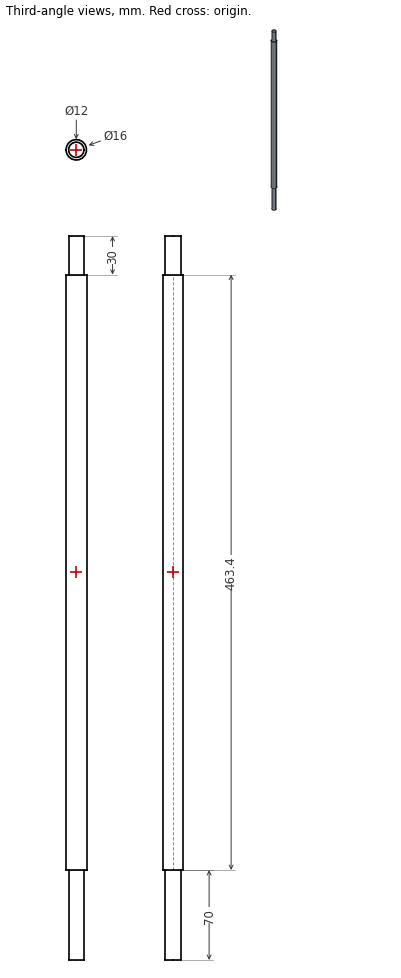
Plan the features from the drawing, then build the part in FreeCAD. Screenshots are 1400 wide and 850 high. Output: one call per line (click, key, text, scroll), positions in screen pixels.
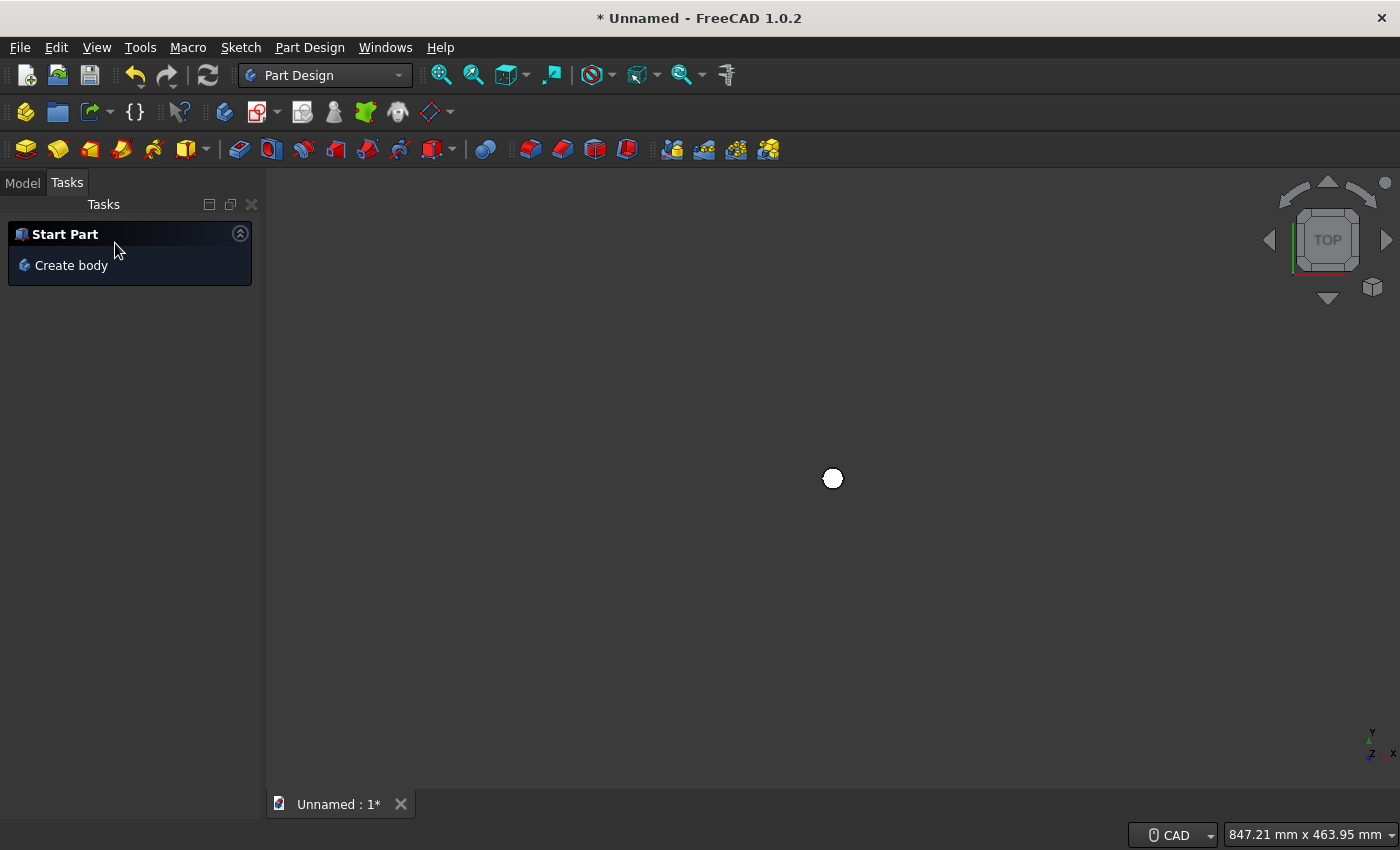
key(v)
key(f)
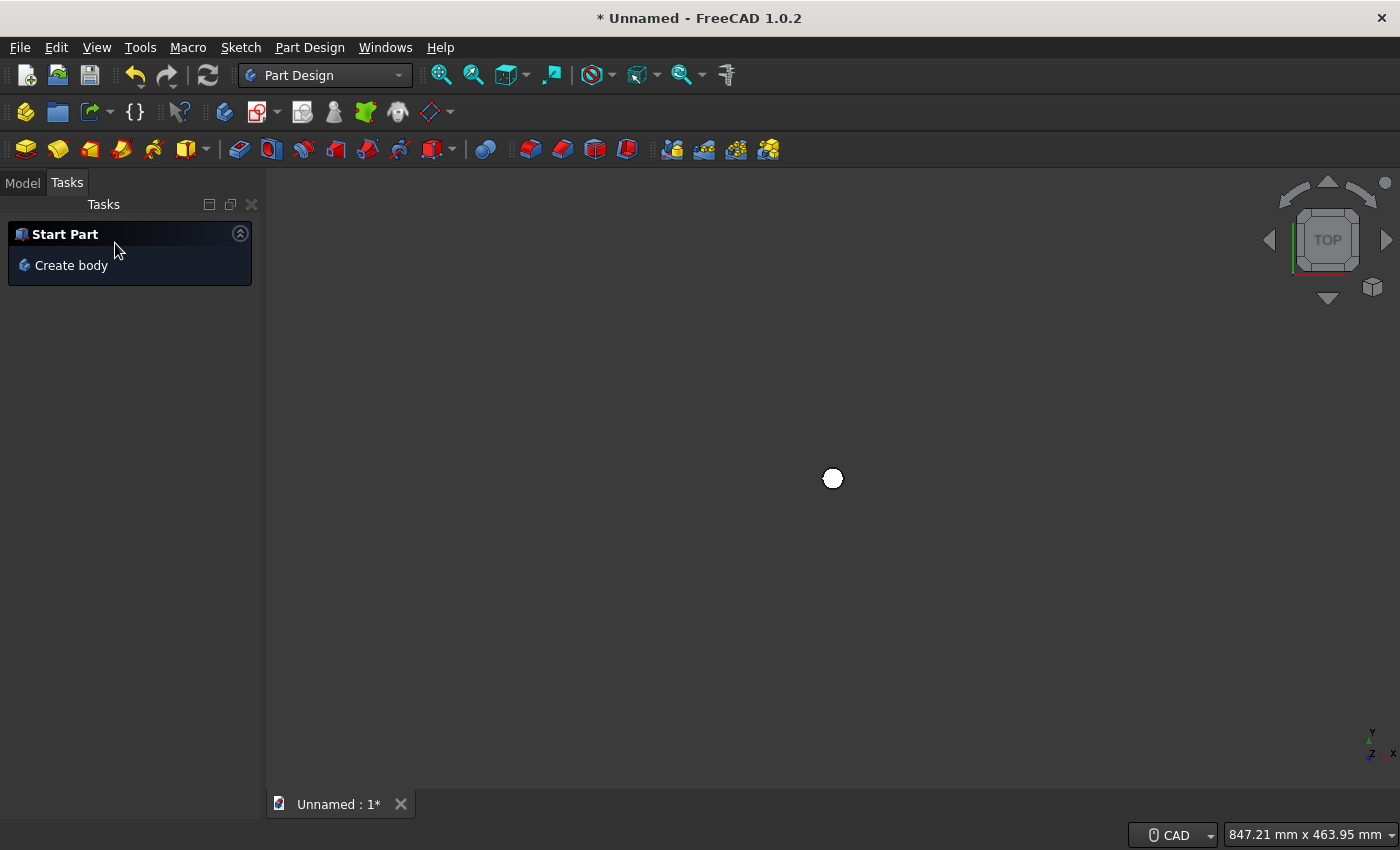
click(833, 477)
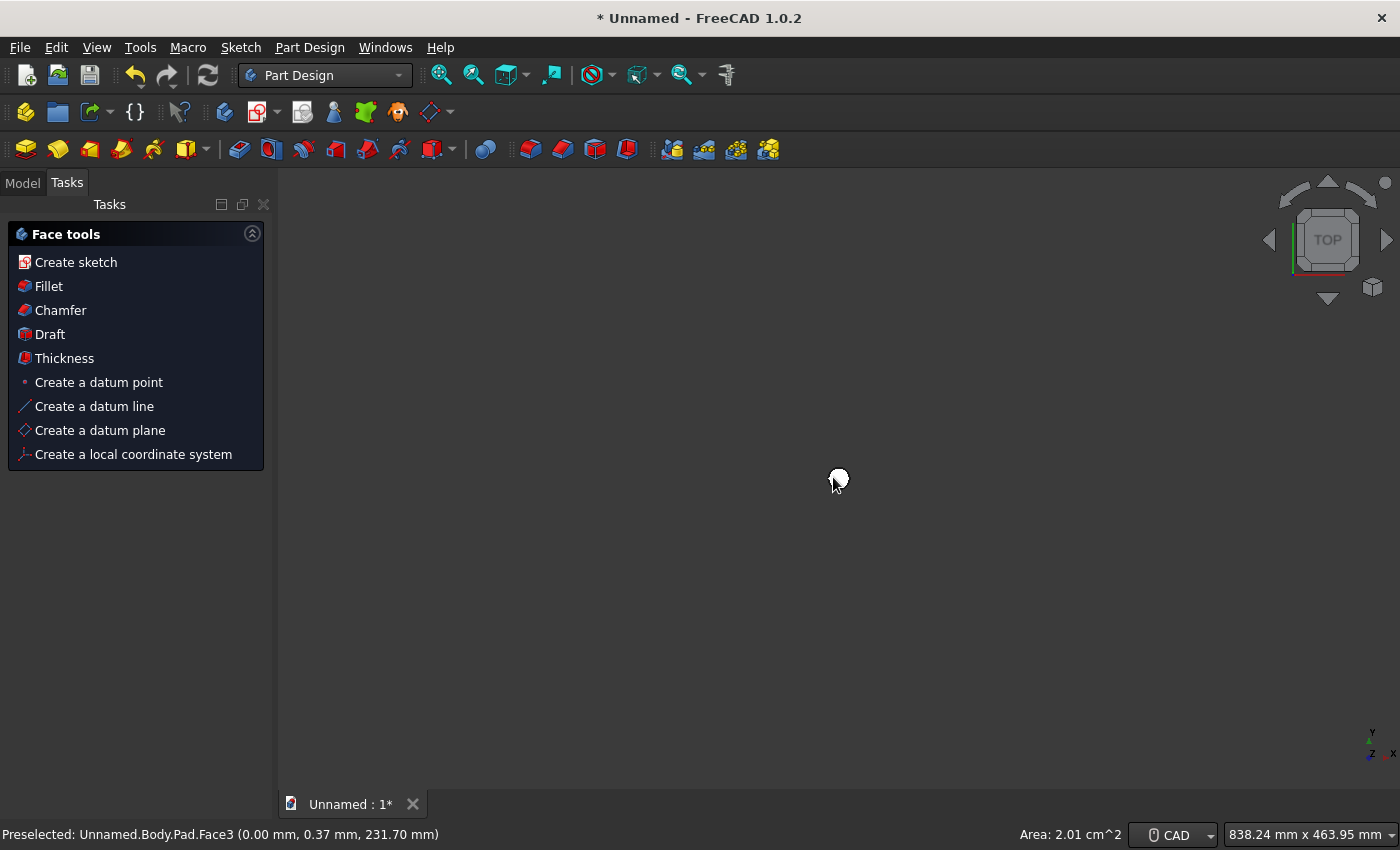
click(258, 112)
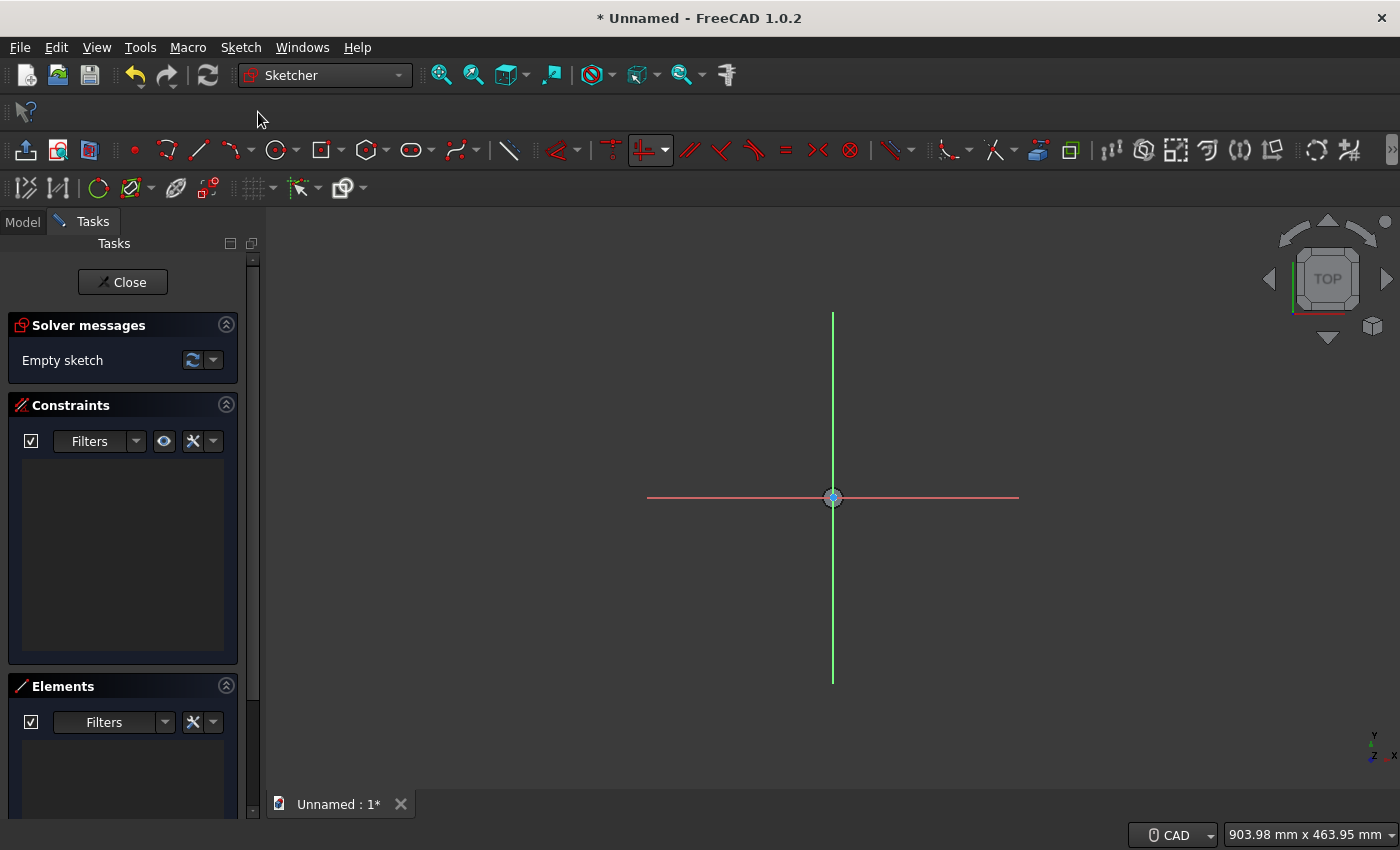
scroll(837, 498, up, 15)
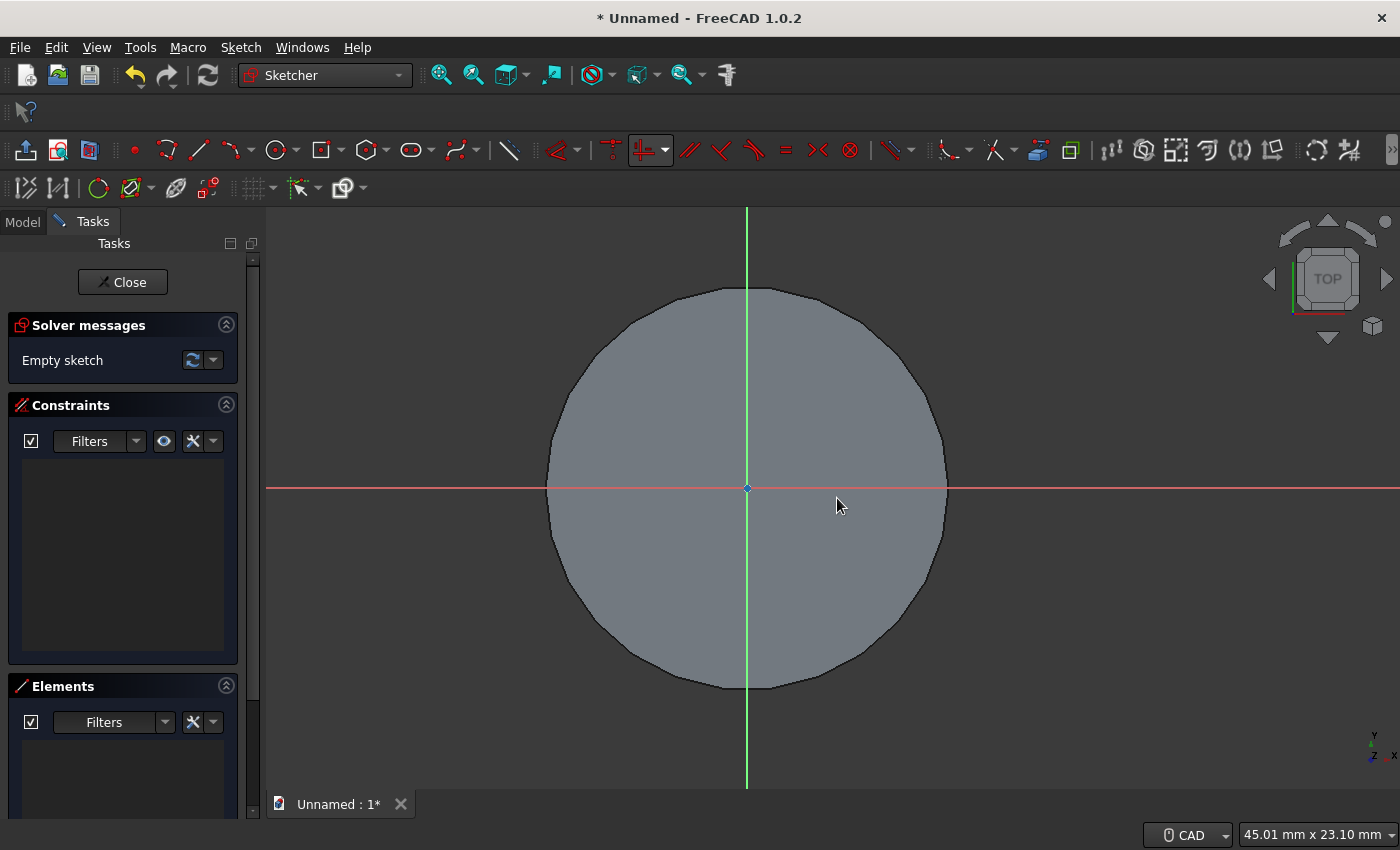
click(276, 150)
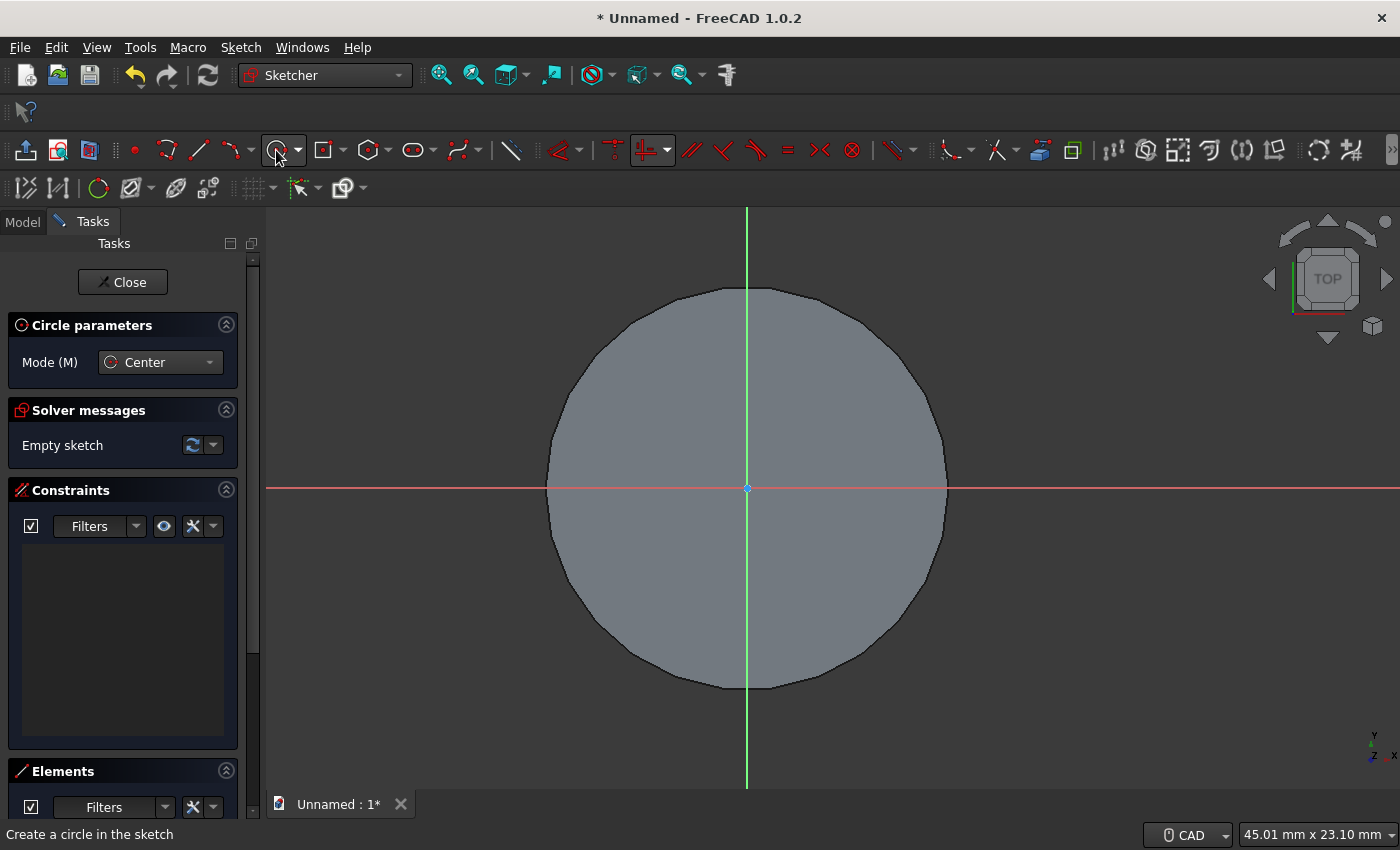
click(747, 488)
click(854, 382)
key(Escape)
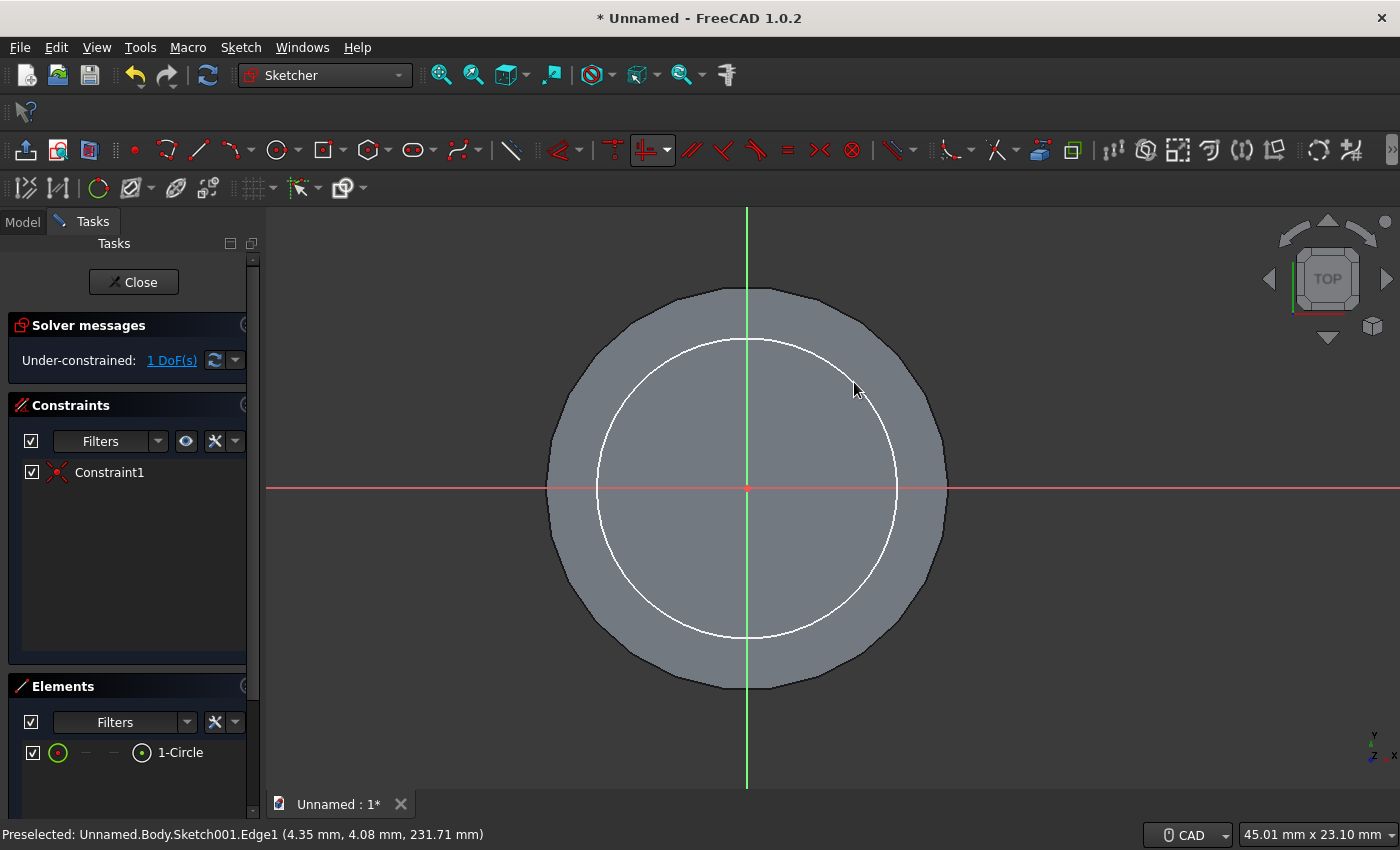
key(d)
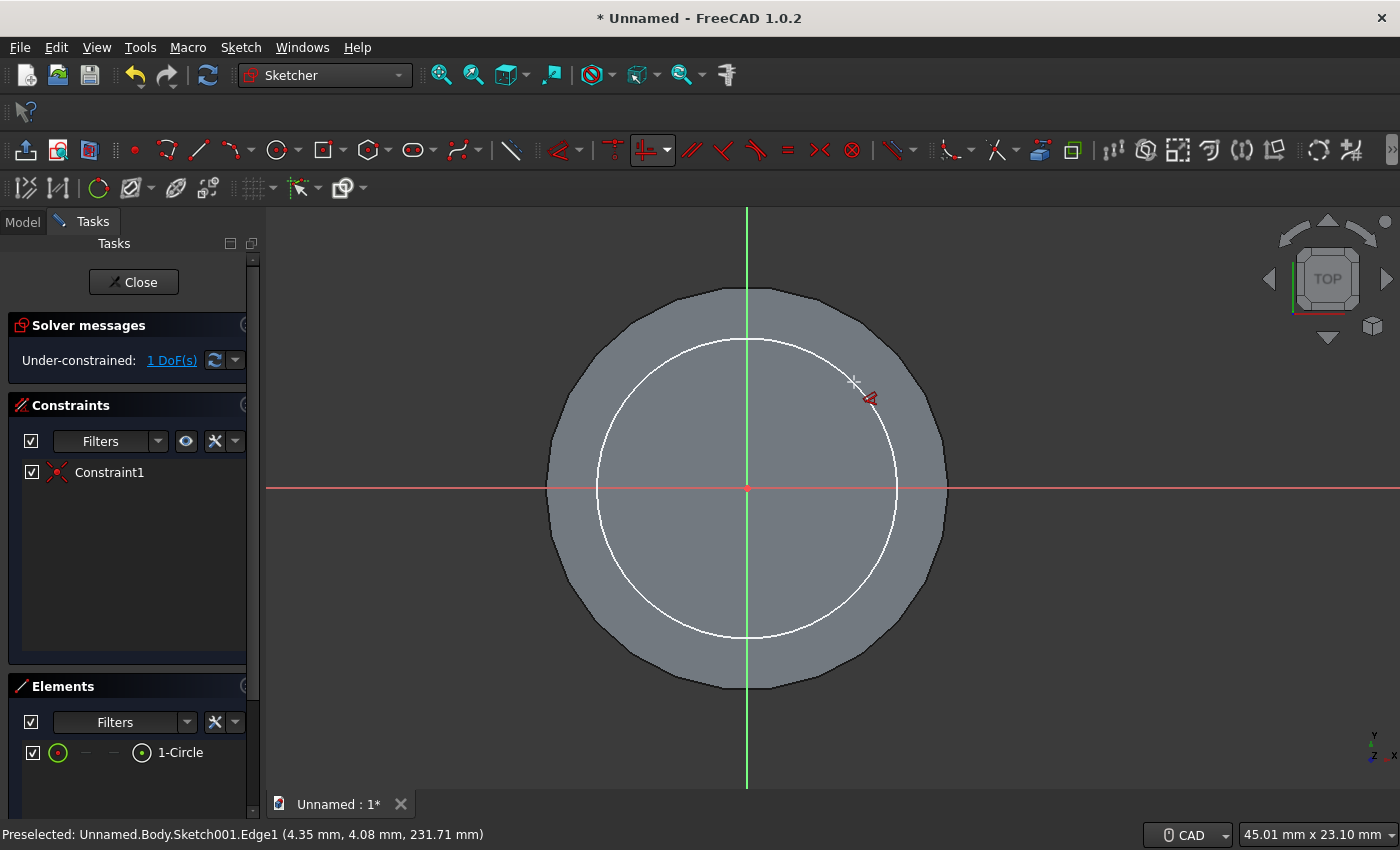
click(853, 382)
click(876, 359)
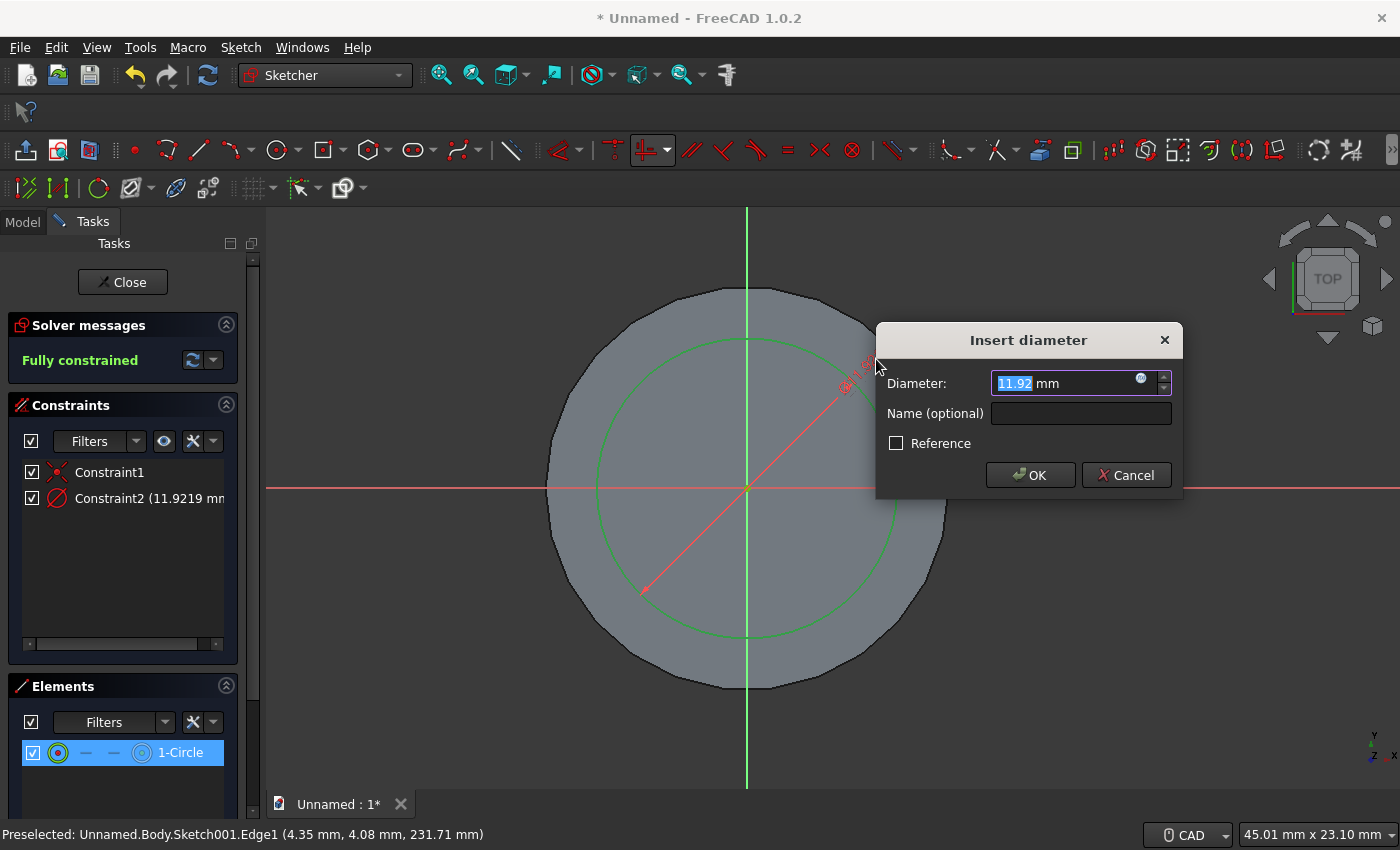
text(12)
key(Return)
key(Escape)